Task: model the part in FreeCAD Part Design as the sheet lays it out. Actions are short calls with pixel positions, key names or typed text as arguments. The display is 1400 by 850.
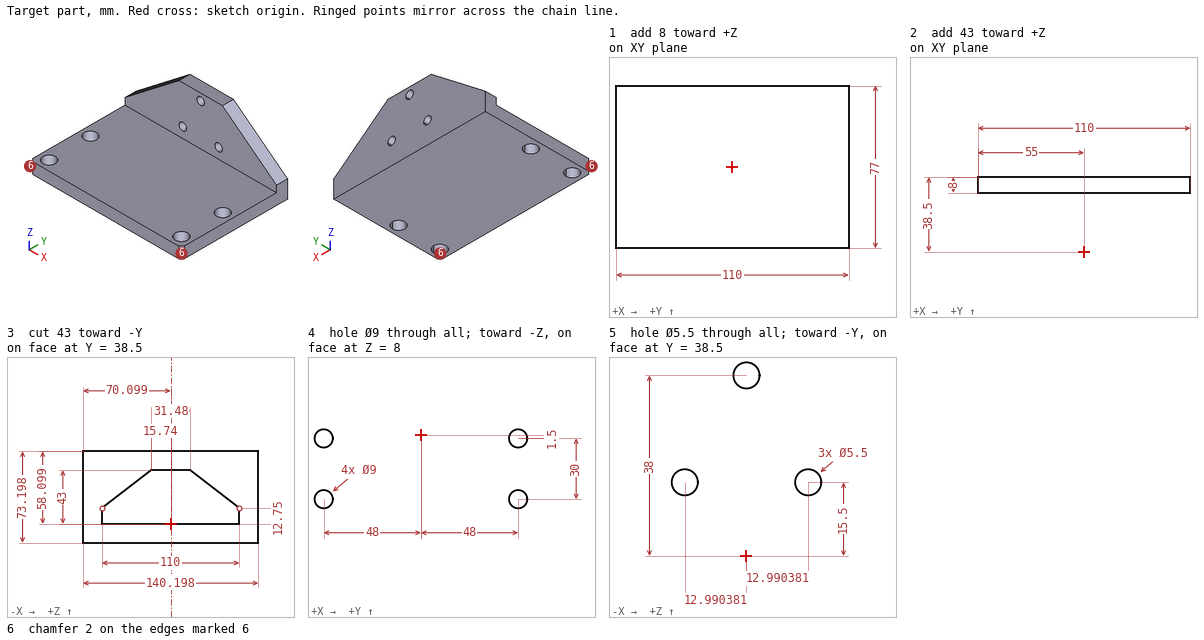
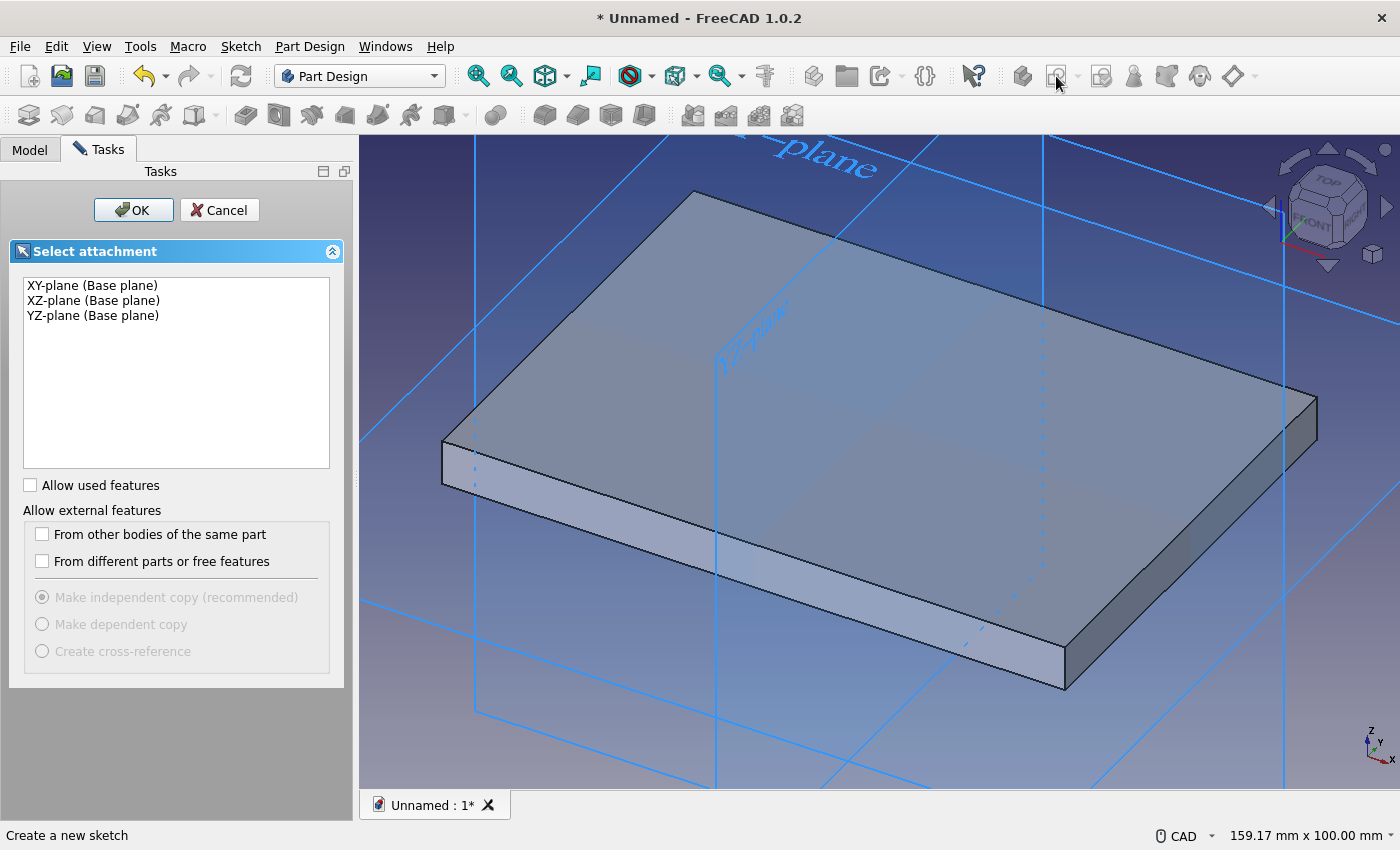
click(84, 286)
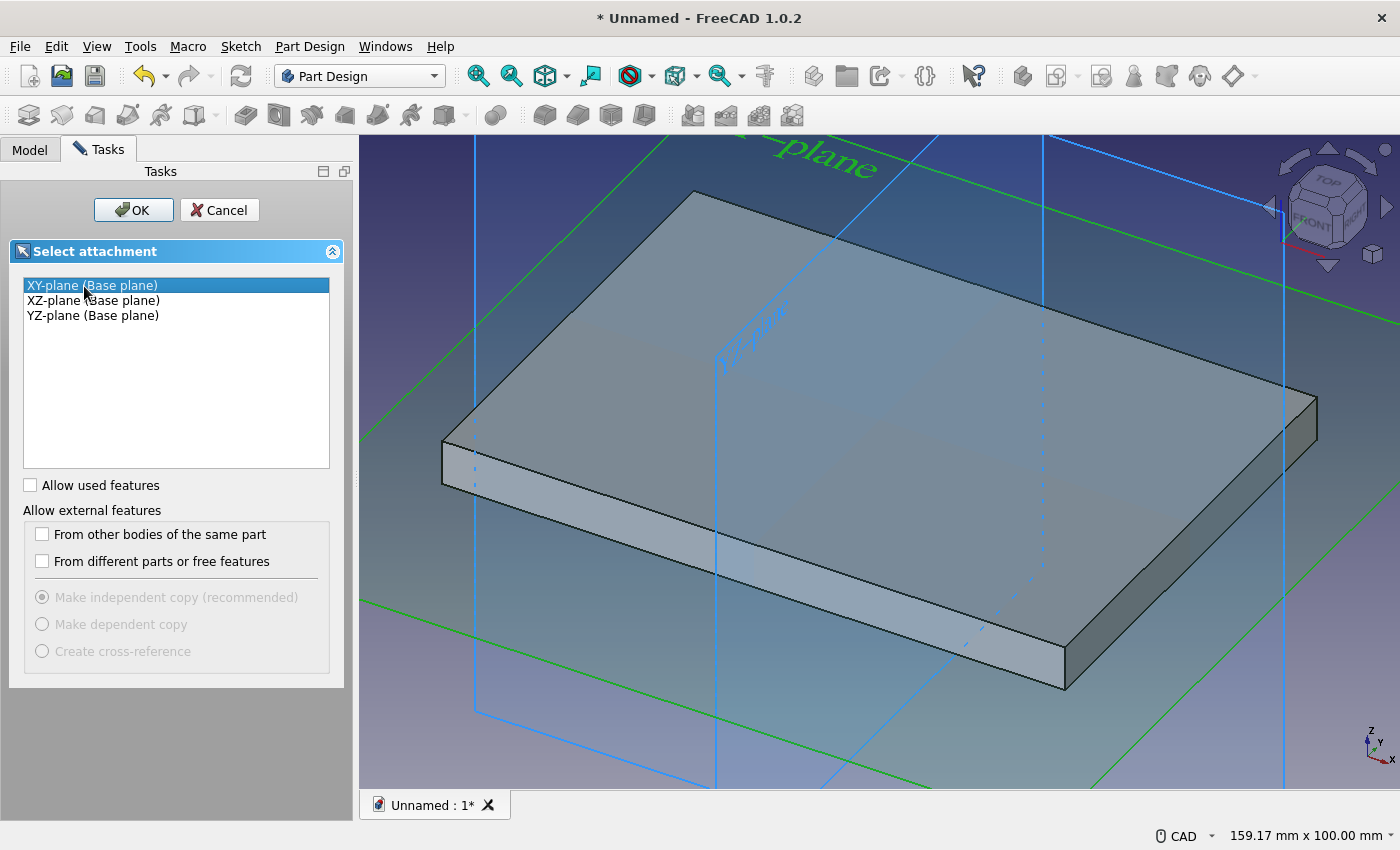
click(134, 210)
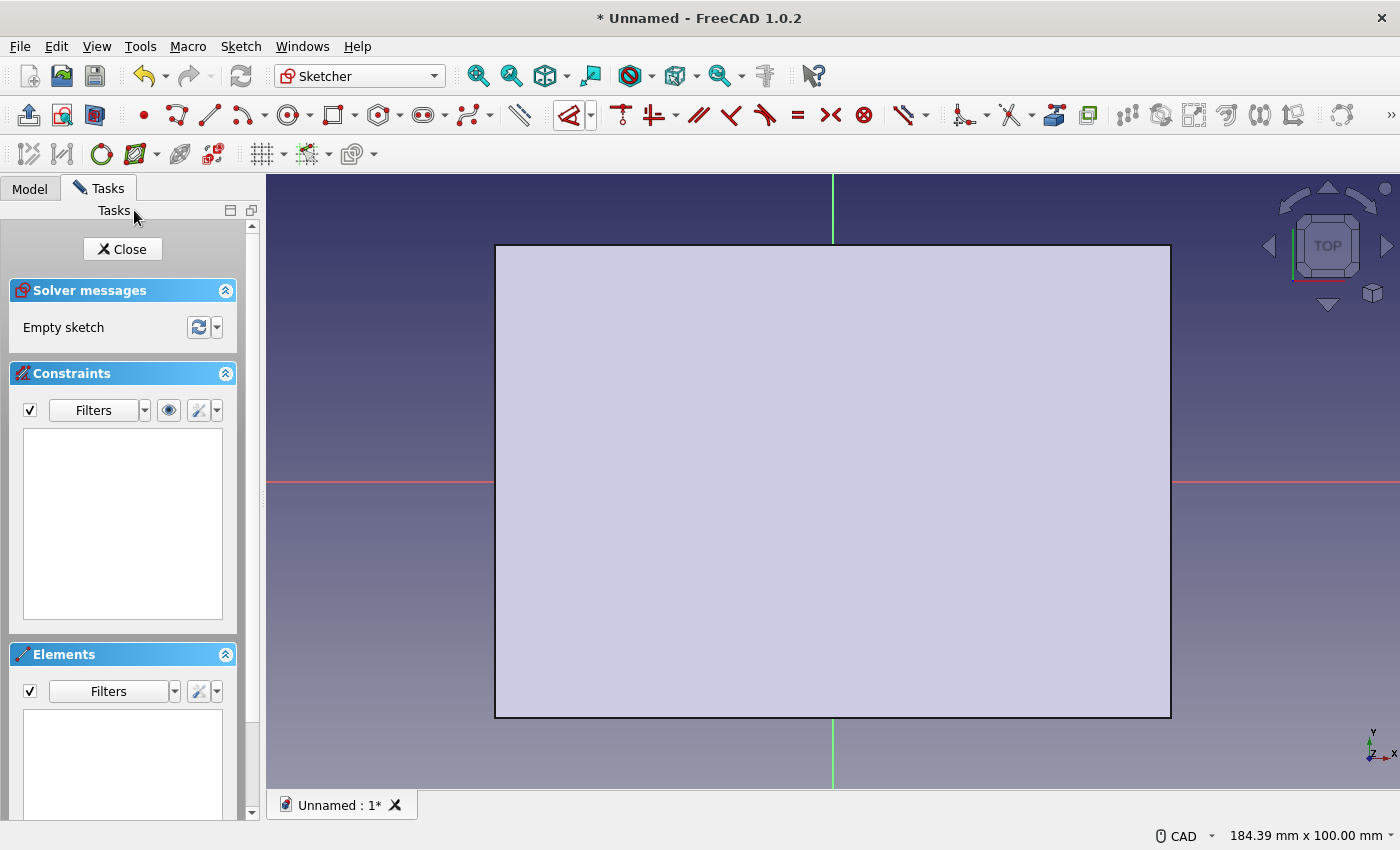
key(q)
key(s)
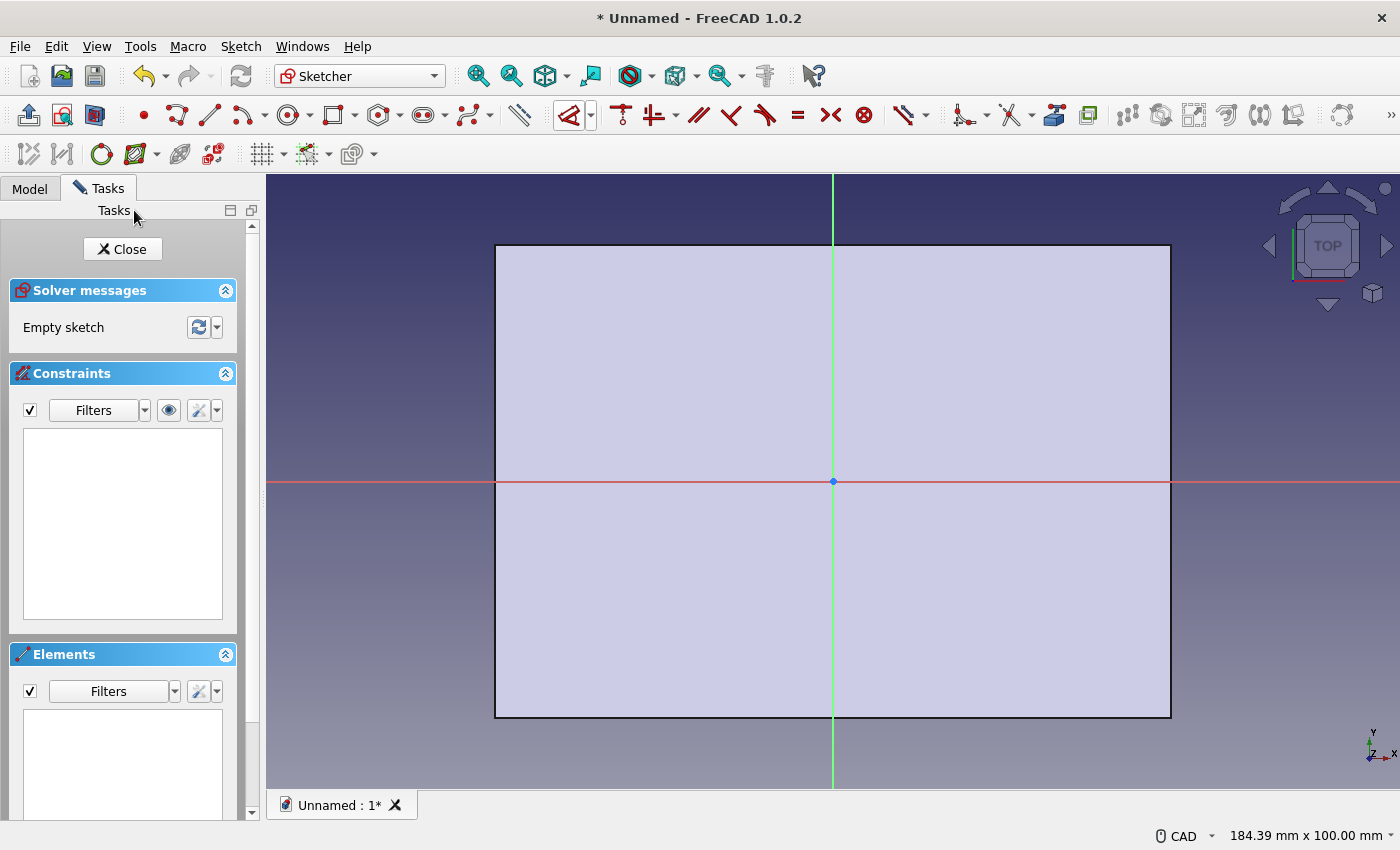
key(g)
key(r)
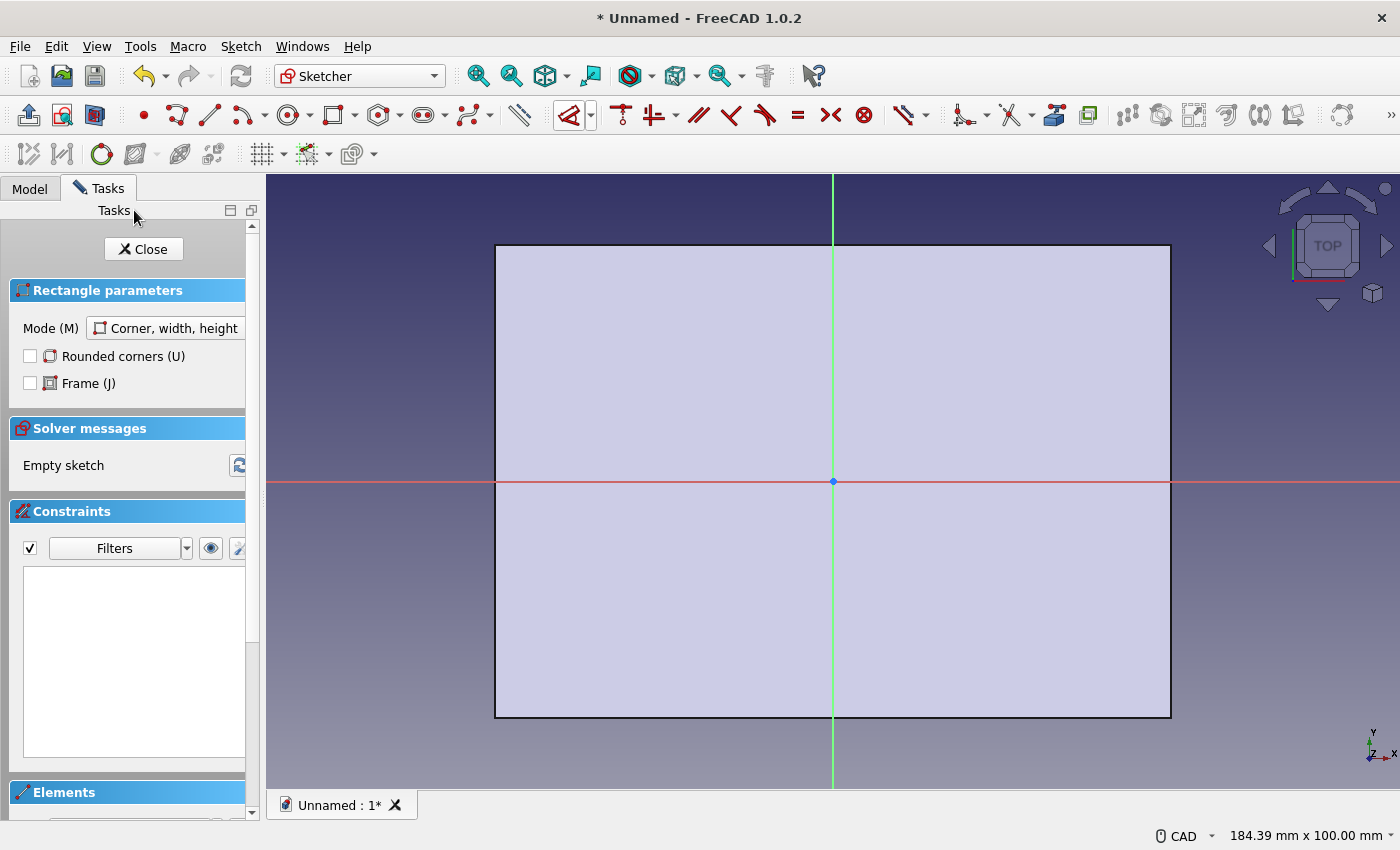
click(495, 245)
click(1171, 294)
key(Escape)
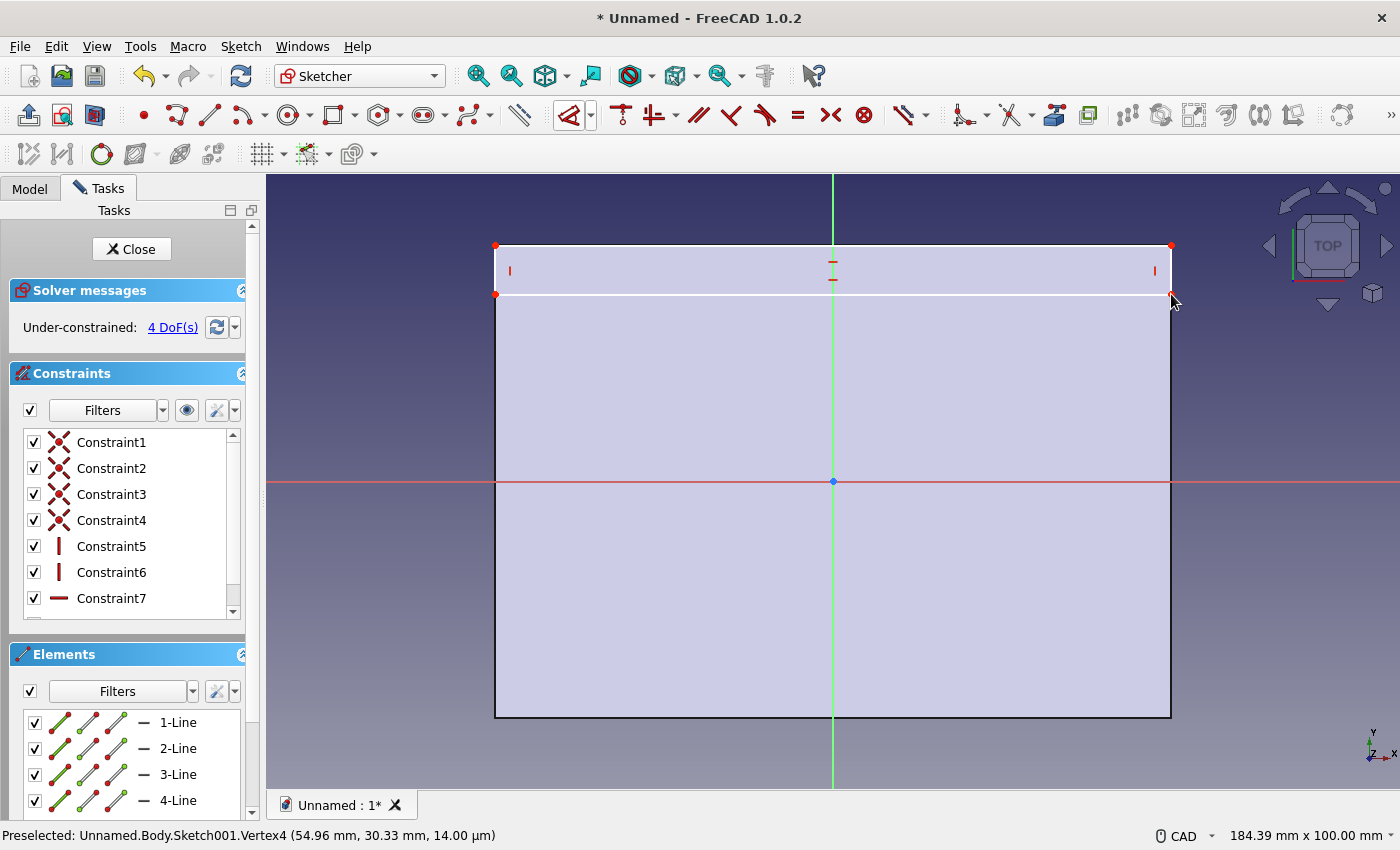
click(495, 261)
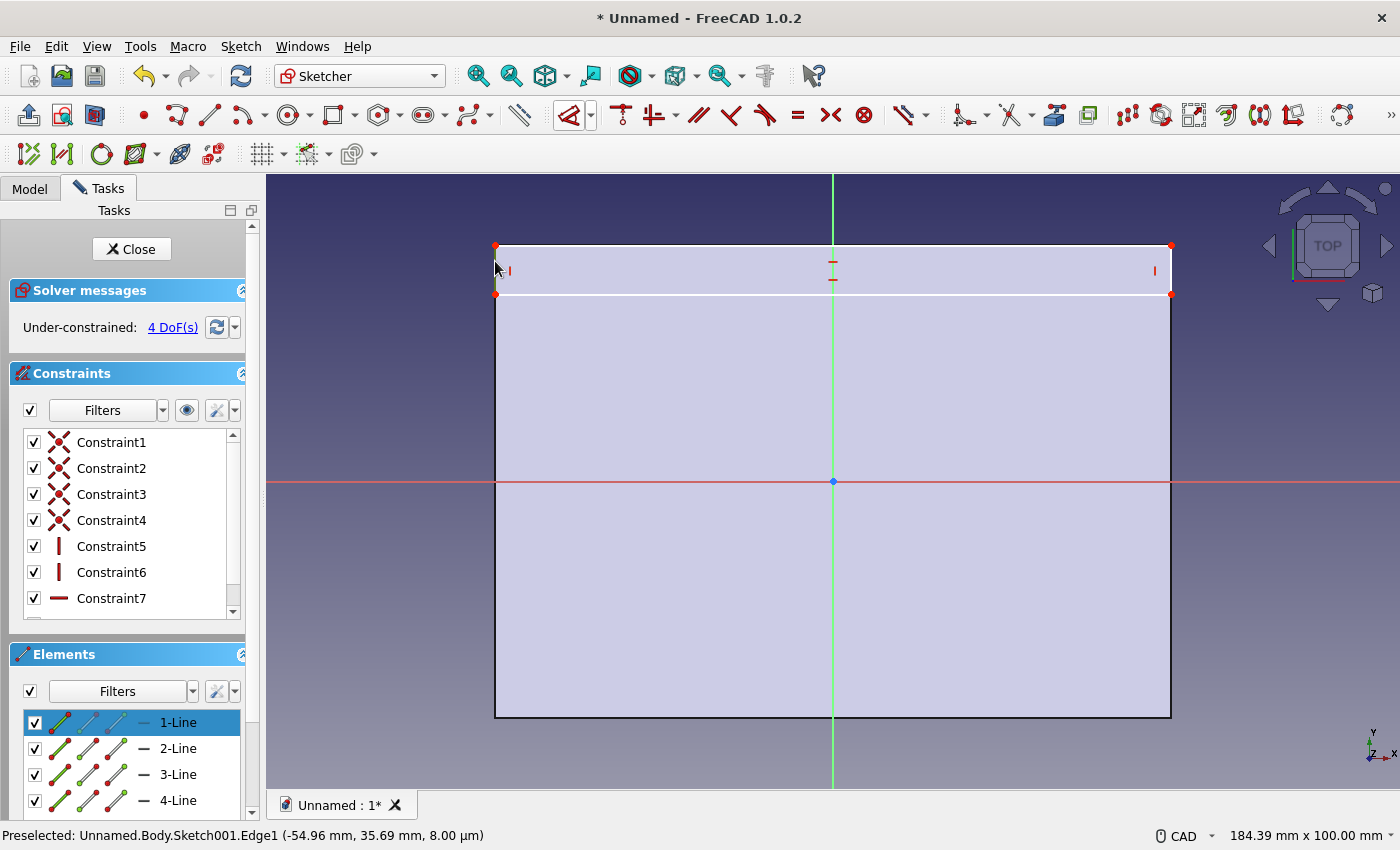
key(i)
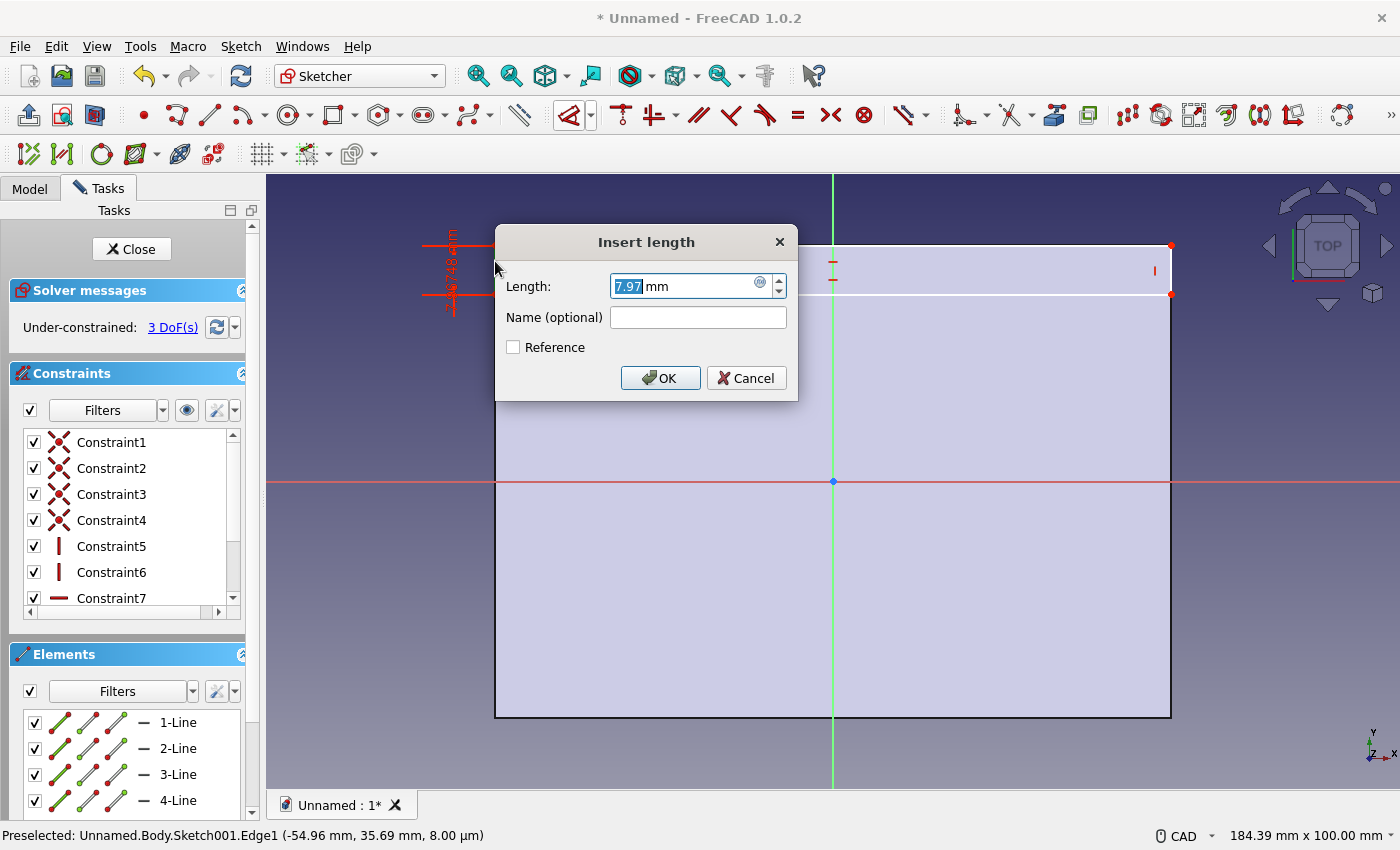
text(8)
key(Return)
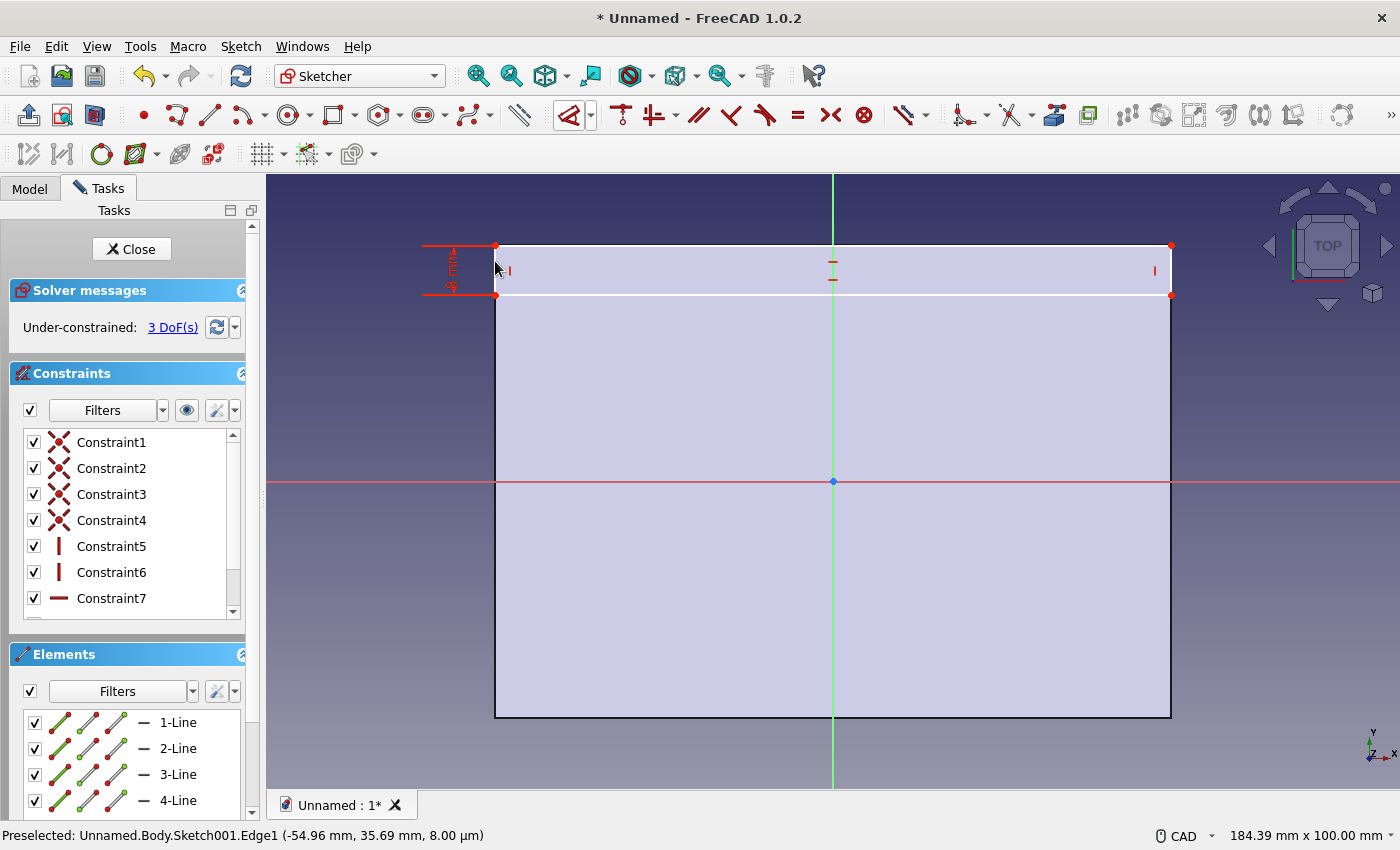
click(698, 295)